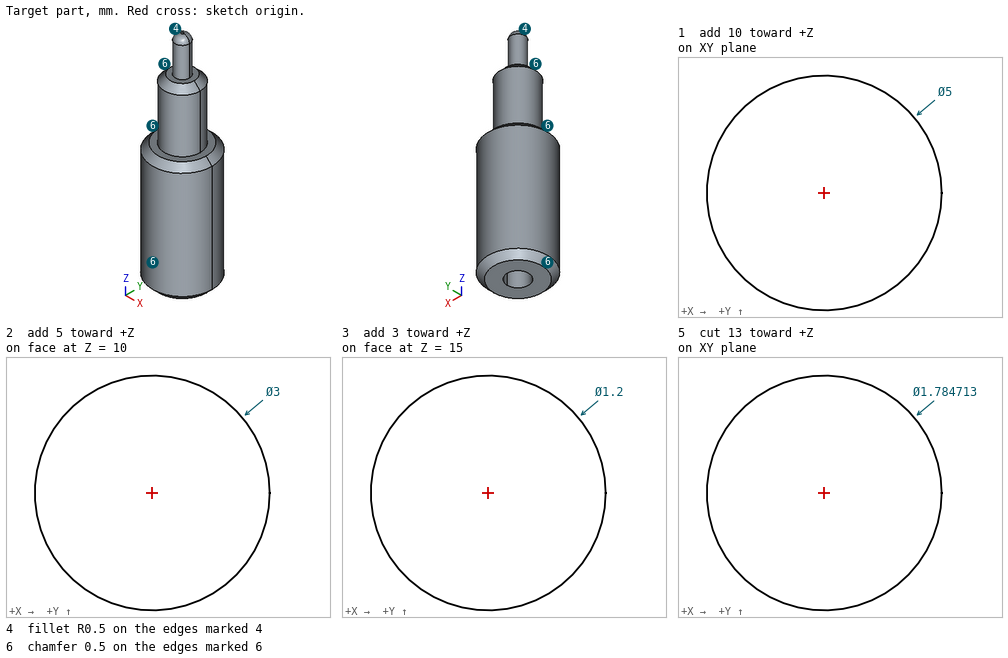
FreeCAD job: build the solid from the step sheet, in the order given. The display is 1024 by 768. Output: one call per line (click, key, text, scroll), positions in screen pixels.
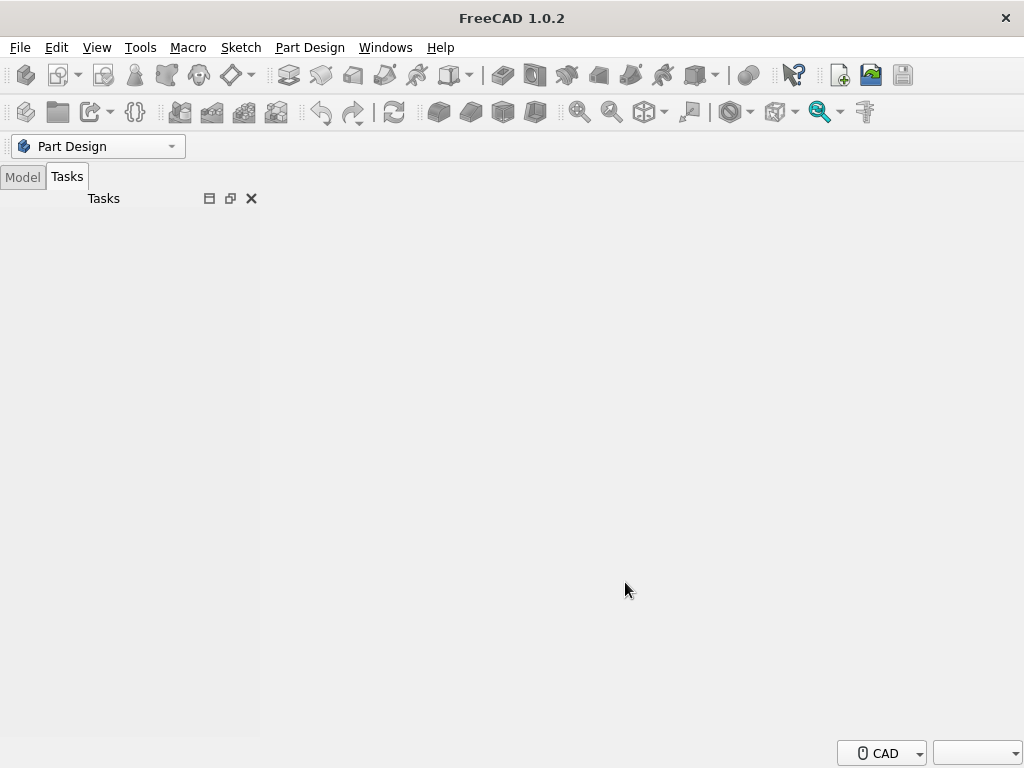
click(840, 76)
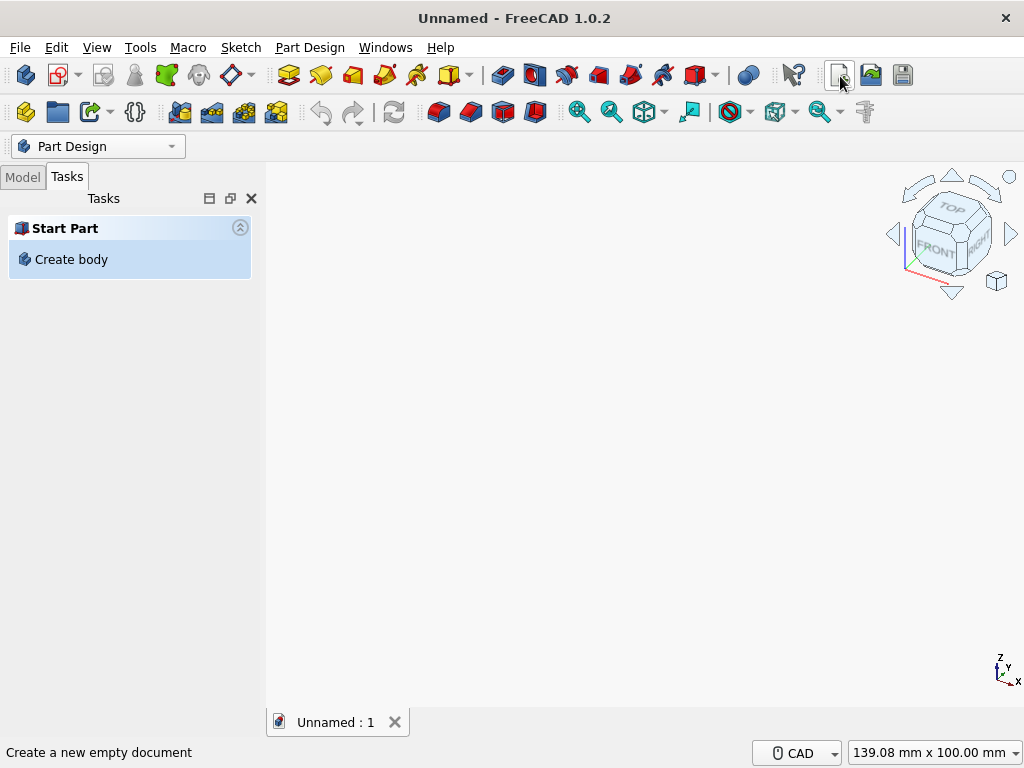
click(58, 76)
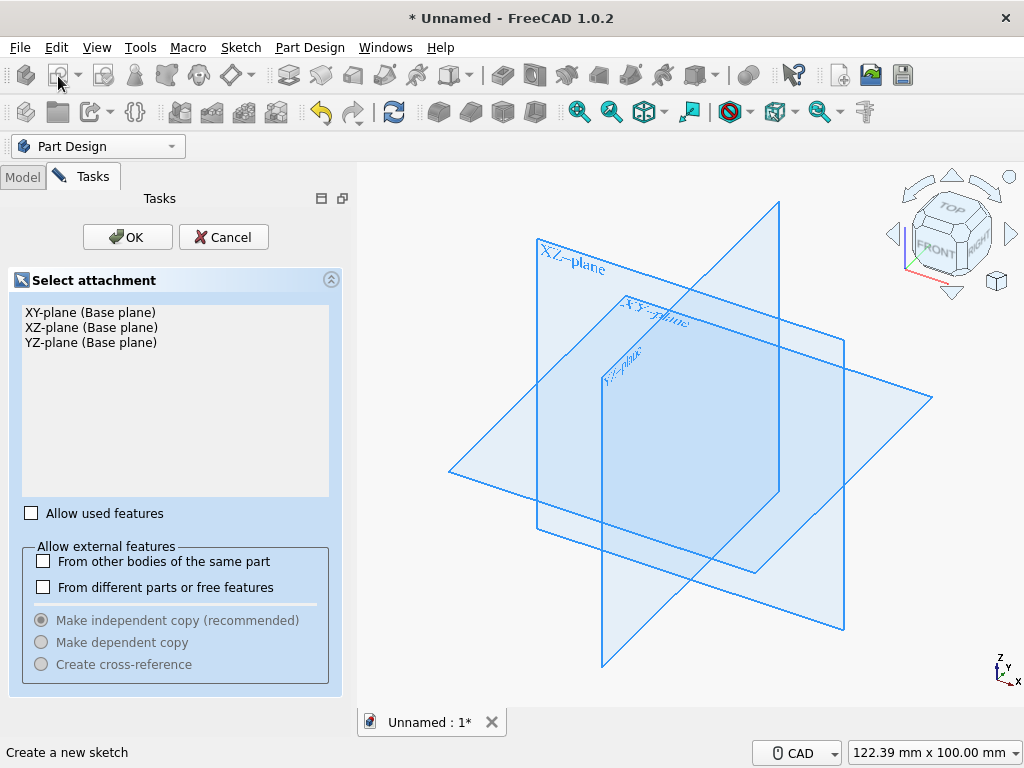
click(82, 312)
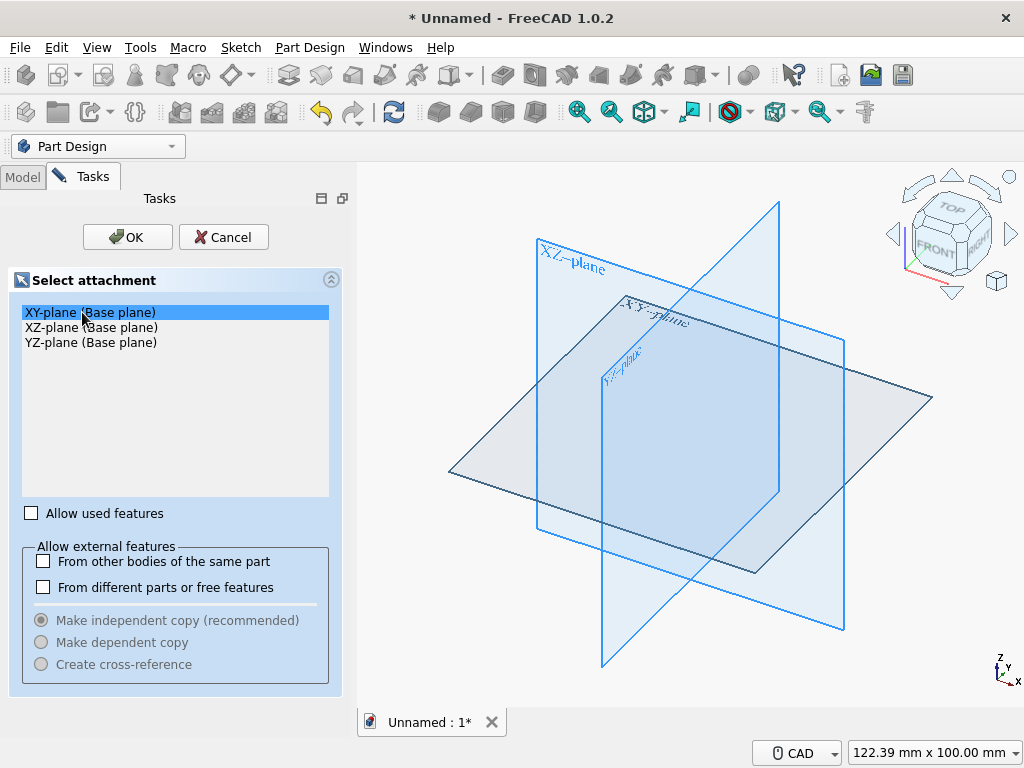
click(128, 237)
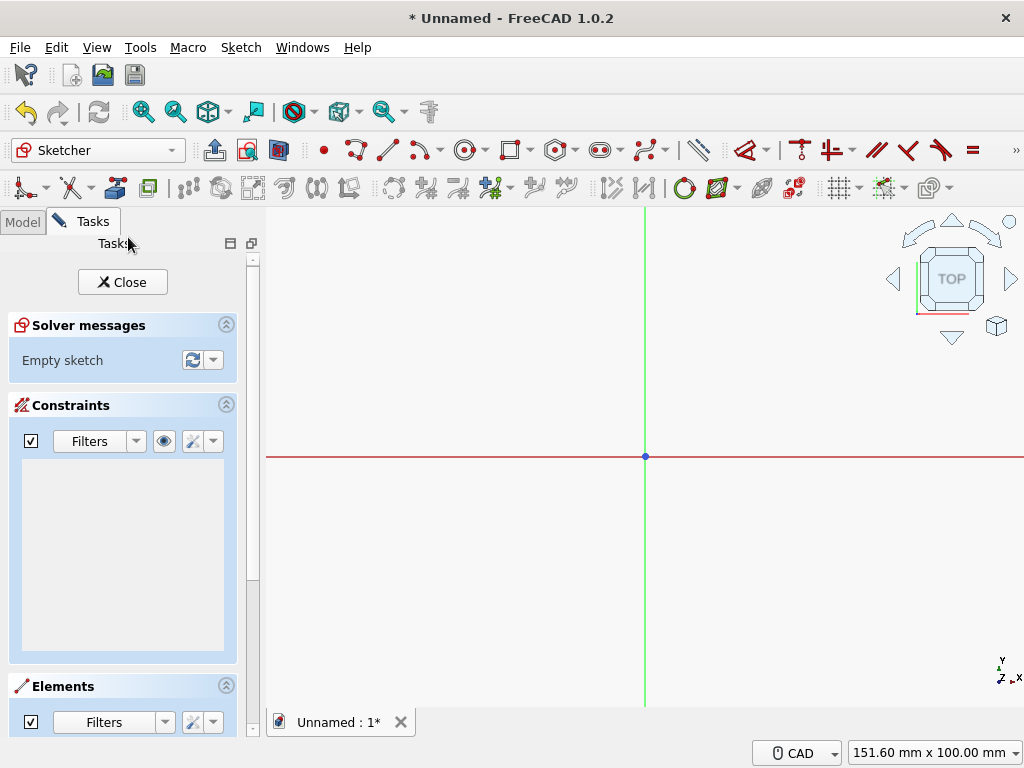
scroll(650, 457, up, 13)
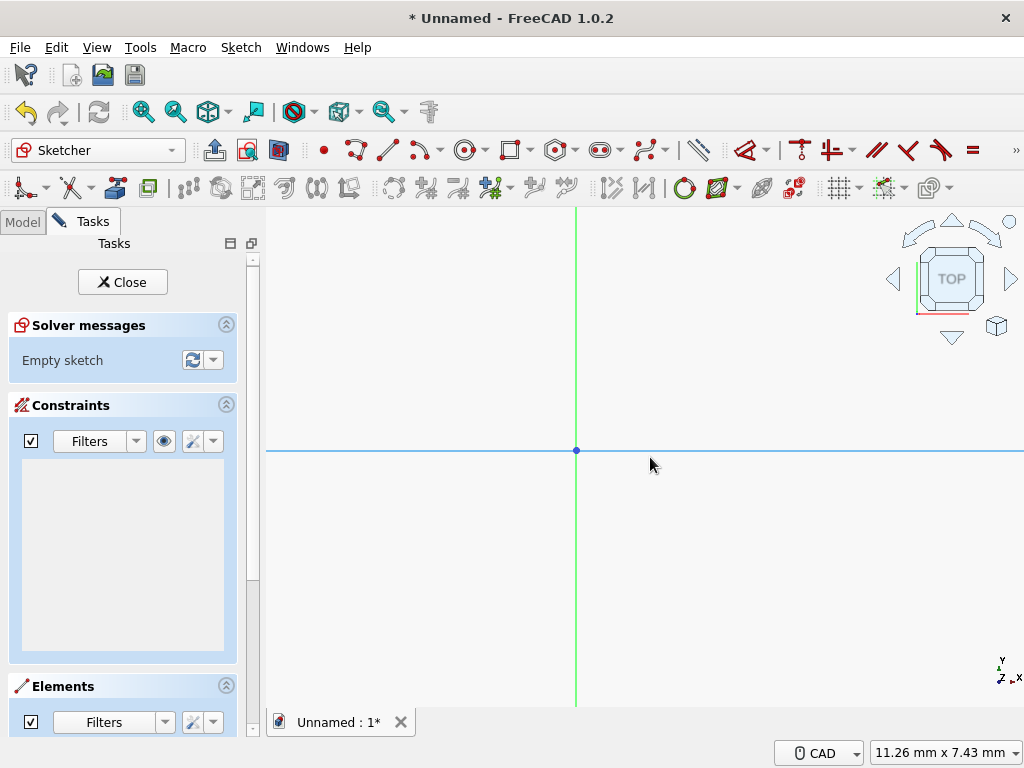
click(466, 150)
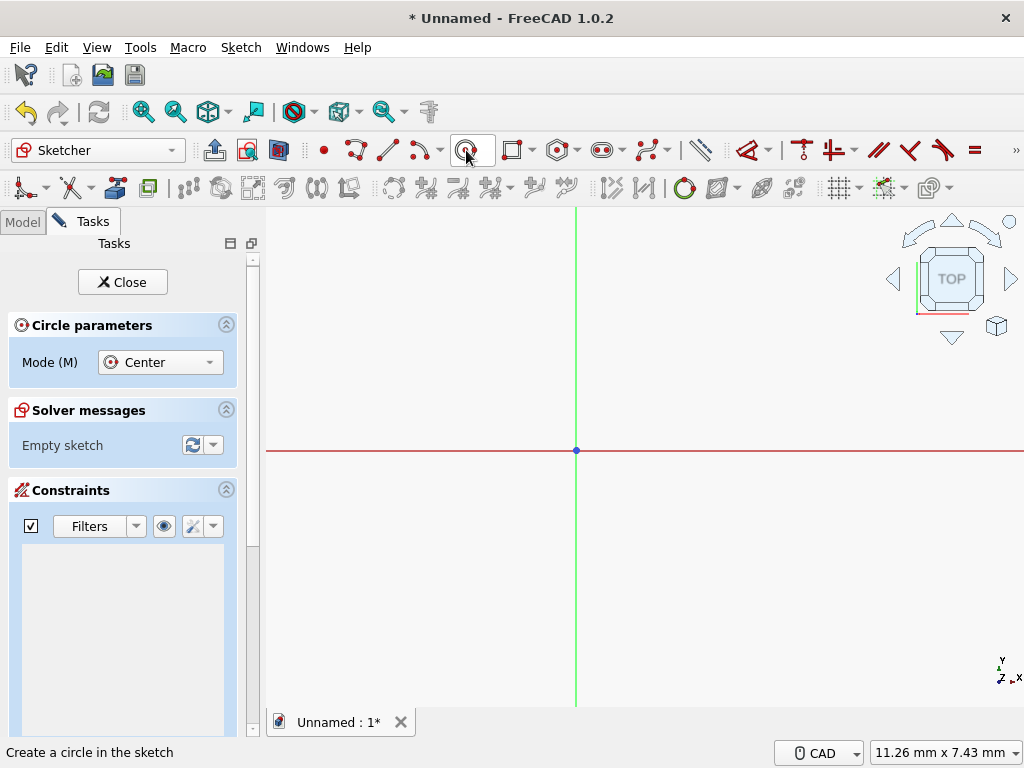
click(576, 451)
move(695, 332)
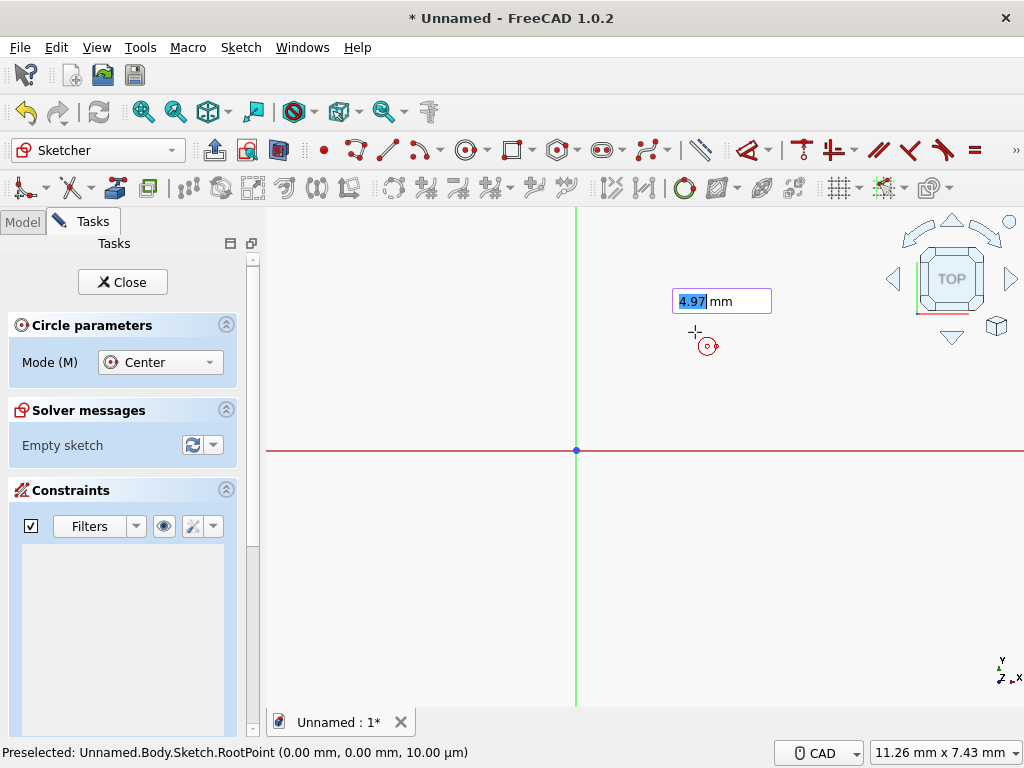
text(5)
key(Return)
key(Escape)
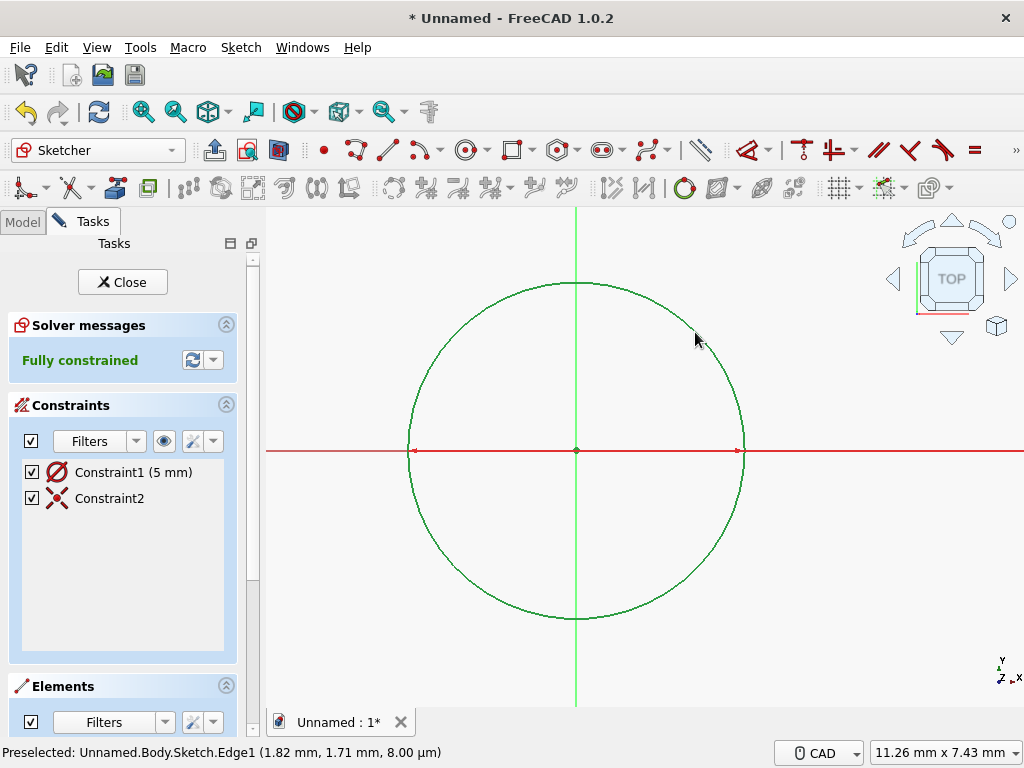
click(123, 282)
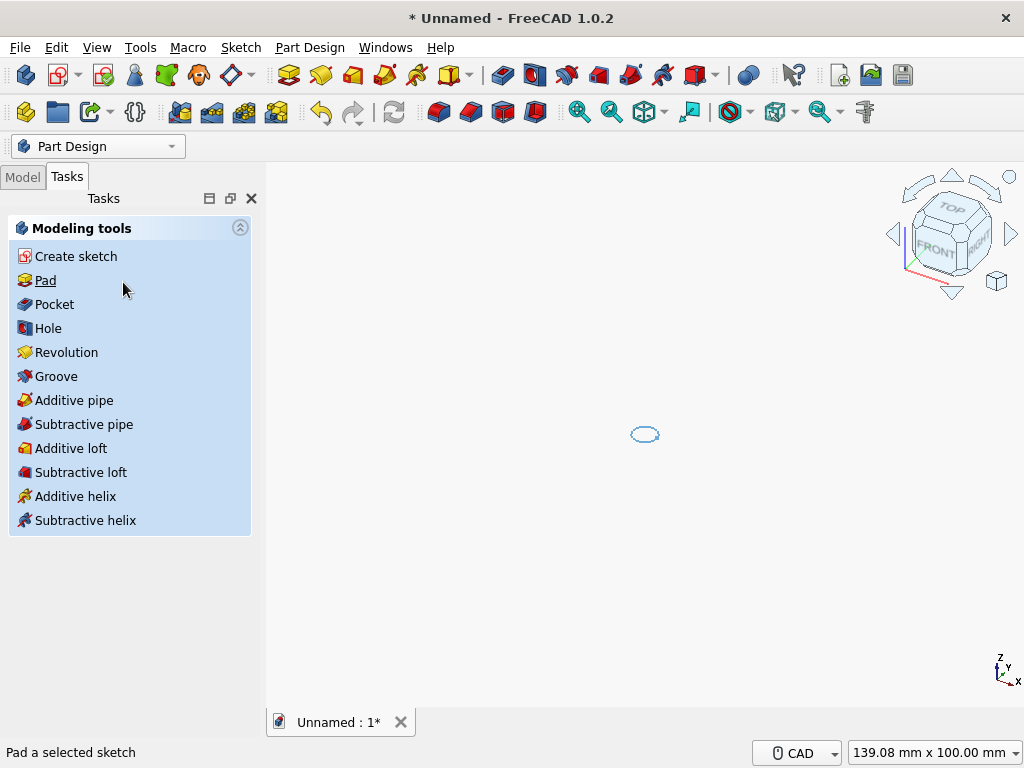
click(290, 76)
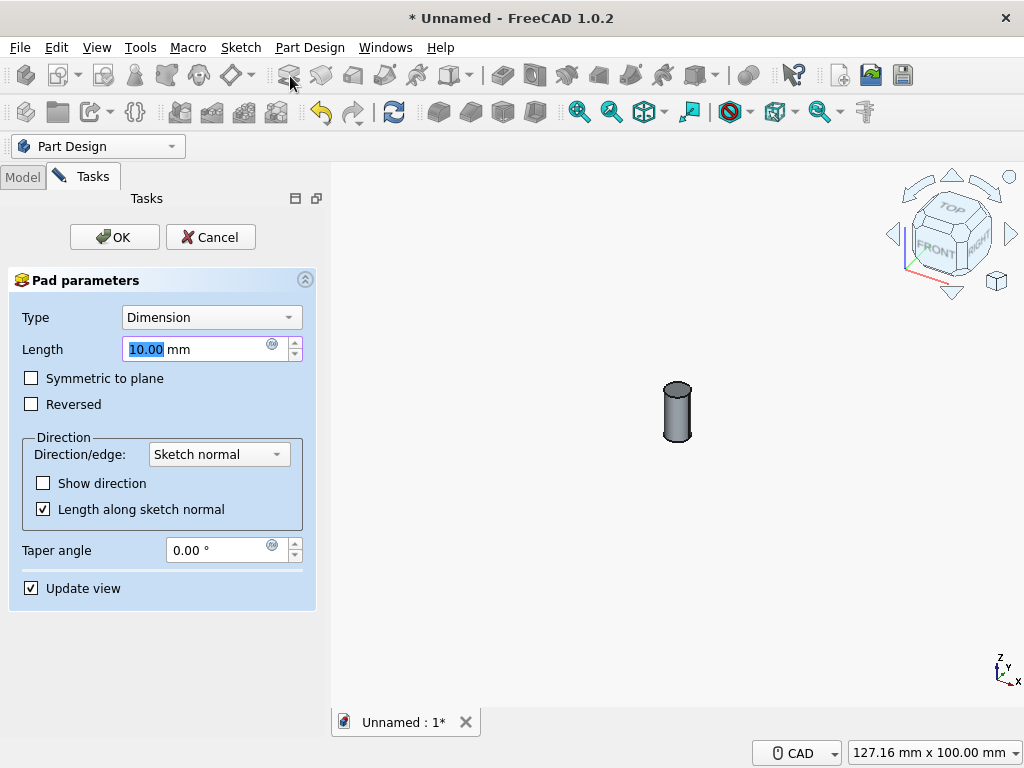
text(10)
key(Tab)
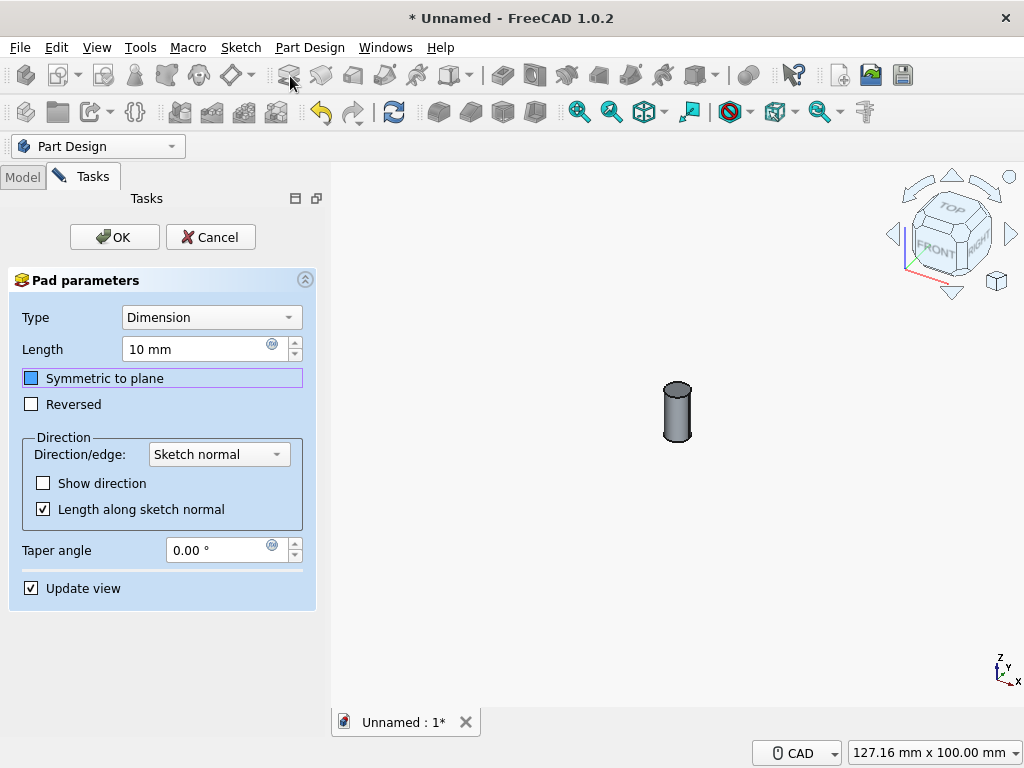
click(115, 237)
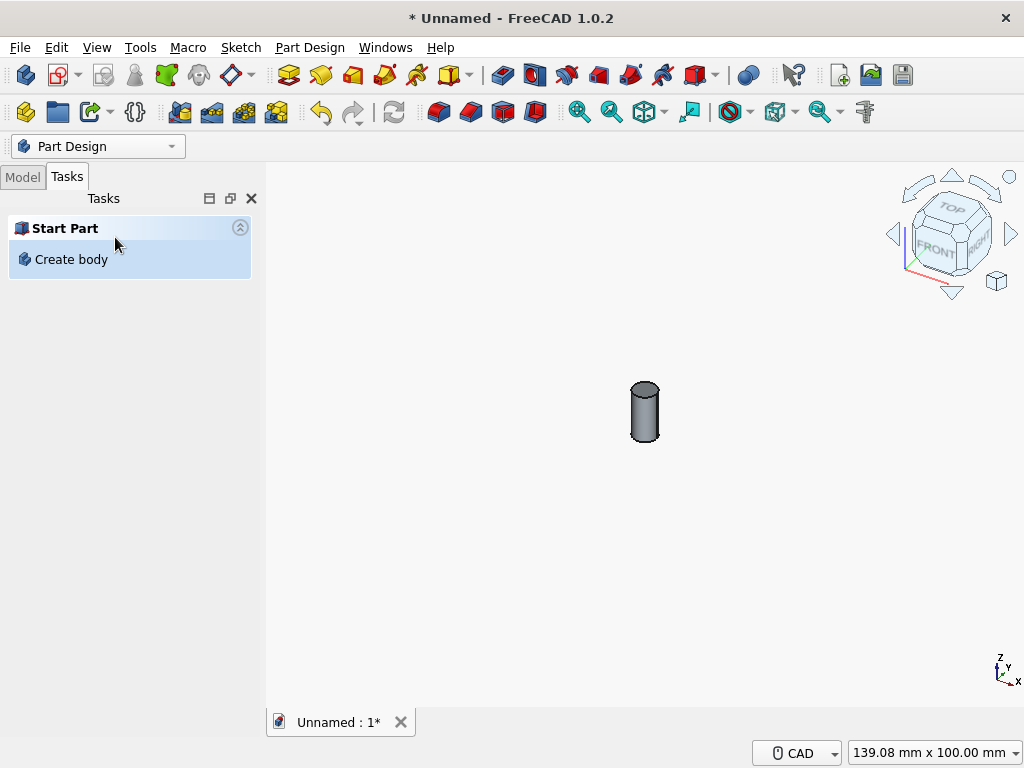
click(580, 112)